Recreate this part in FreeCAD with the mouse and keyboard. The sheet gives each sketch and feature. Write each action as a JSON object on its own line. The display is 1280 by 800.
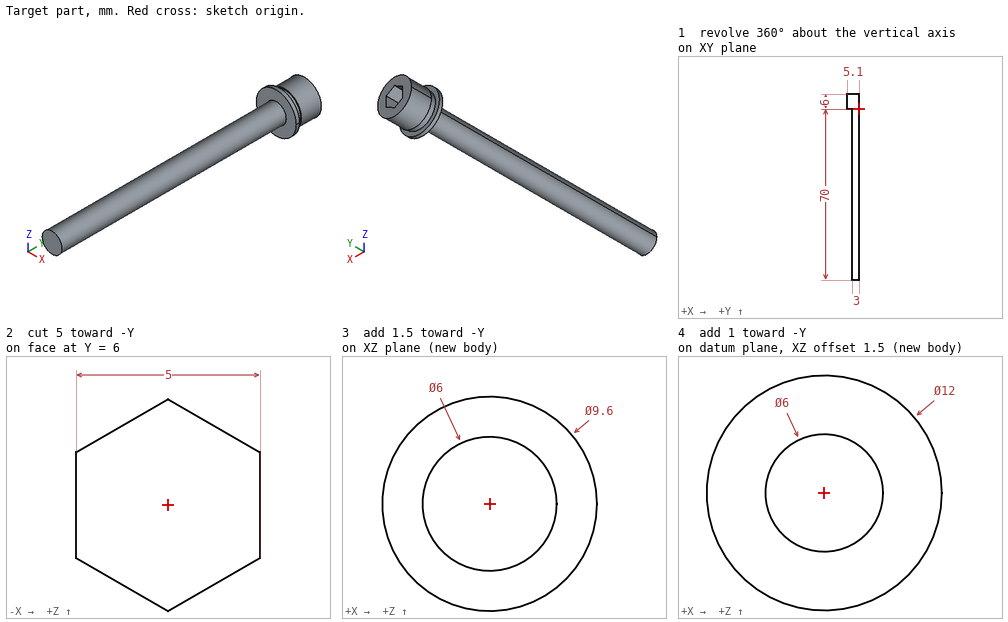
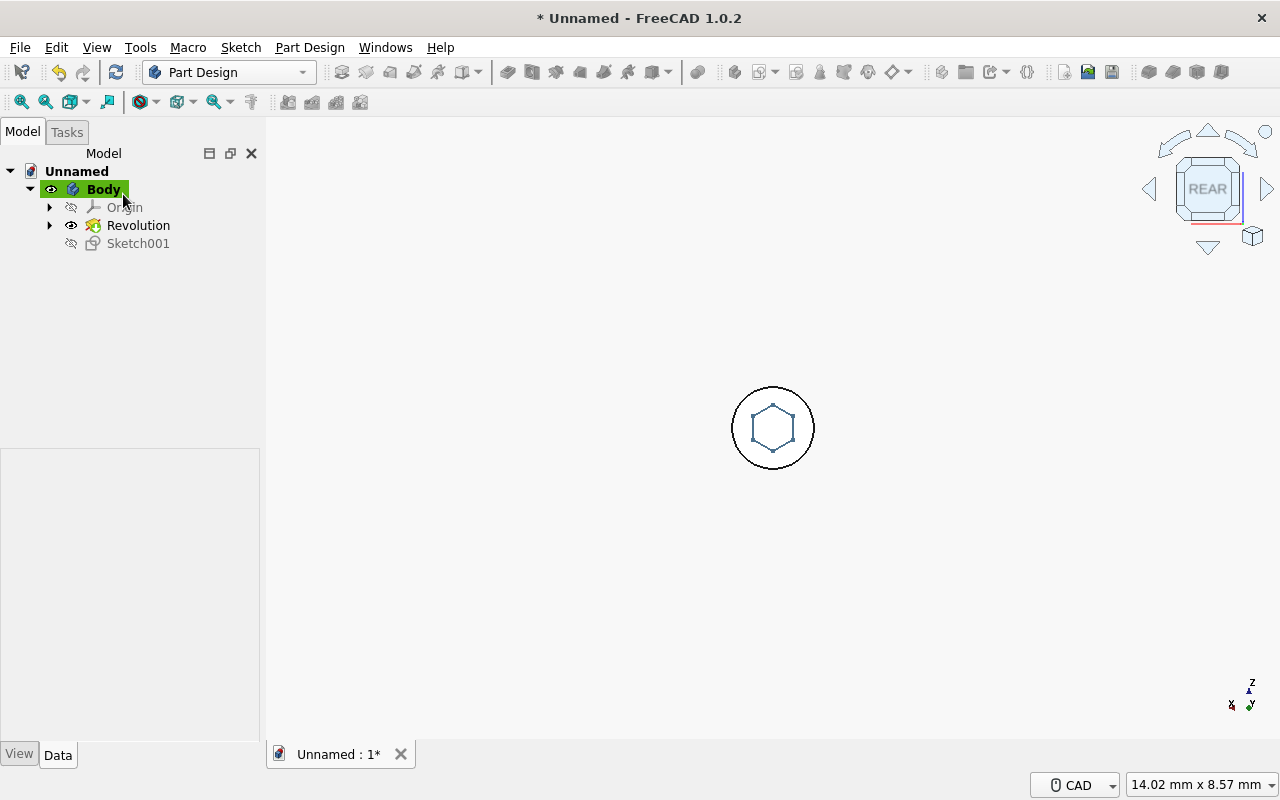
{"action": "left_click", "coordinate": [508, 72]}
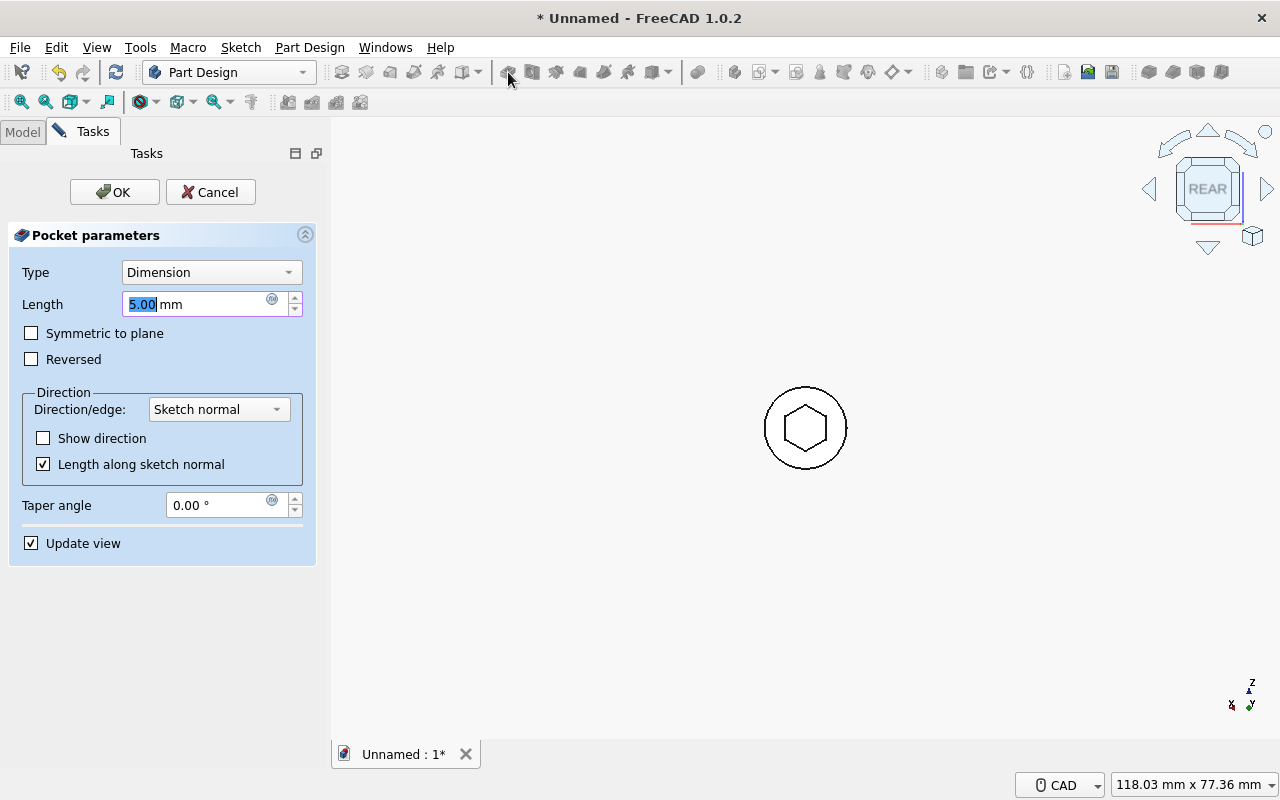
{"action": "type", "text": "5"}
{"action": "key", "text": "Tab"}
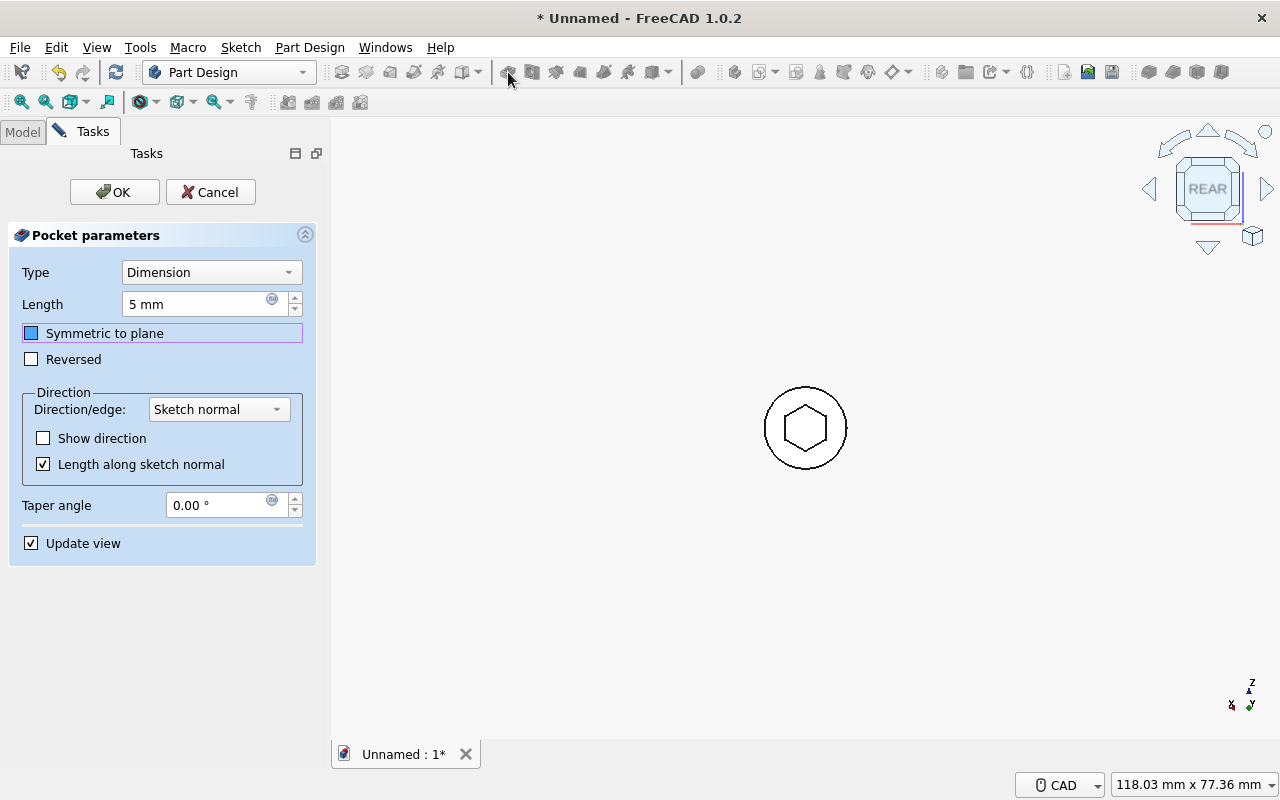
{"action": "left_click", "coordinate": [115, 192]}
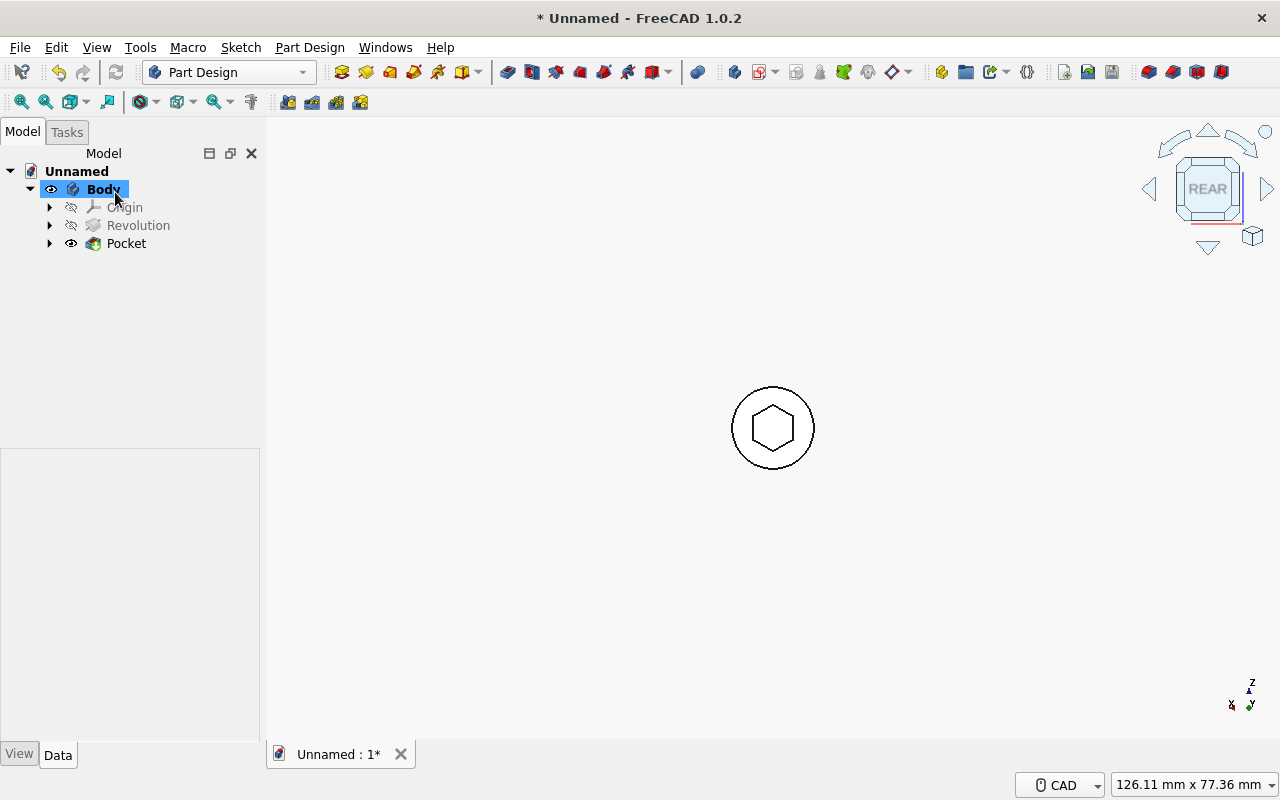
{"action": "key", "text": "v f"}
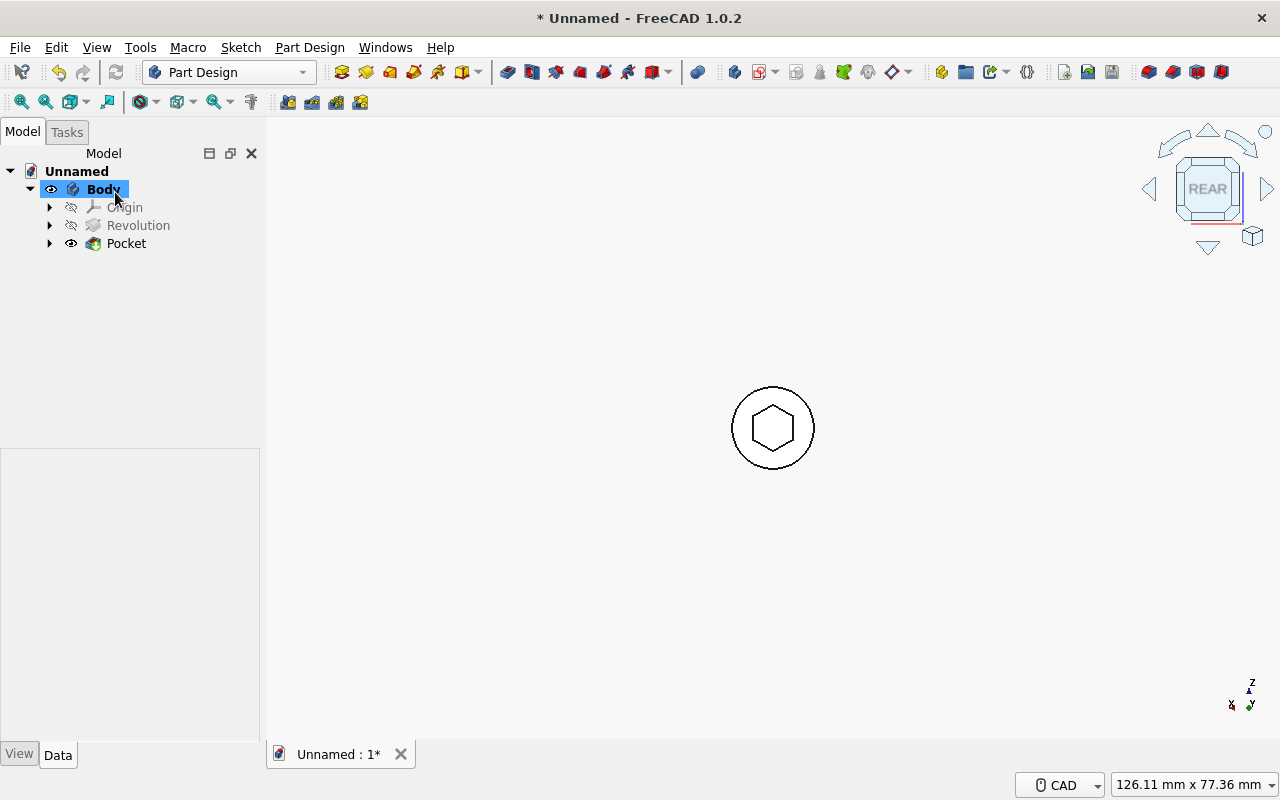
{"action": "left_click", "coordinate": [736, 72]}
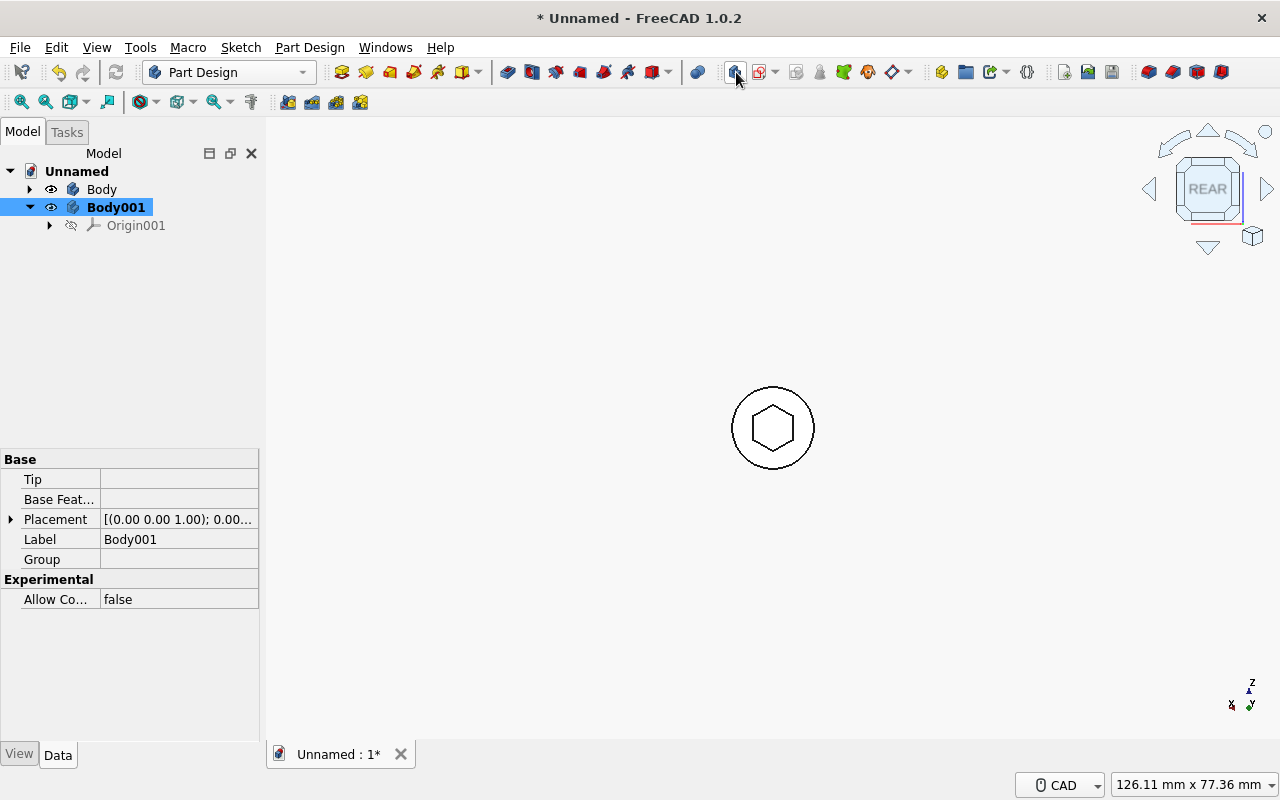
{"action": "left_click", "coordinate": [306, 699]}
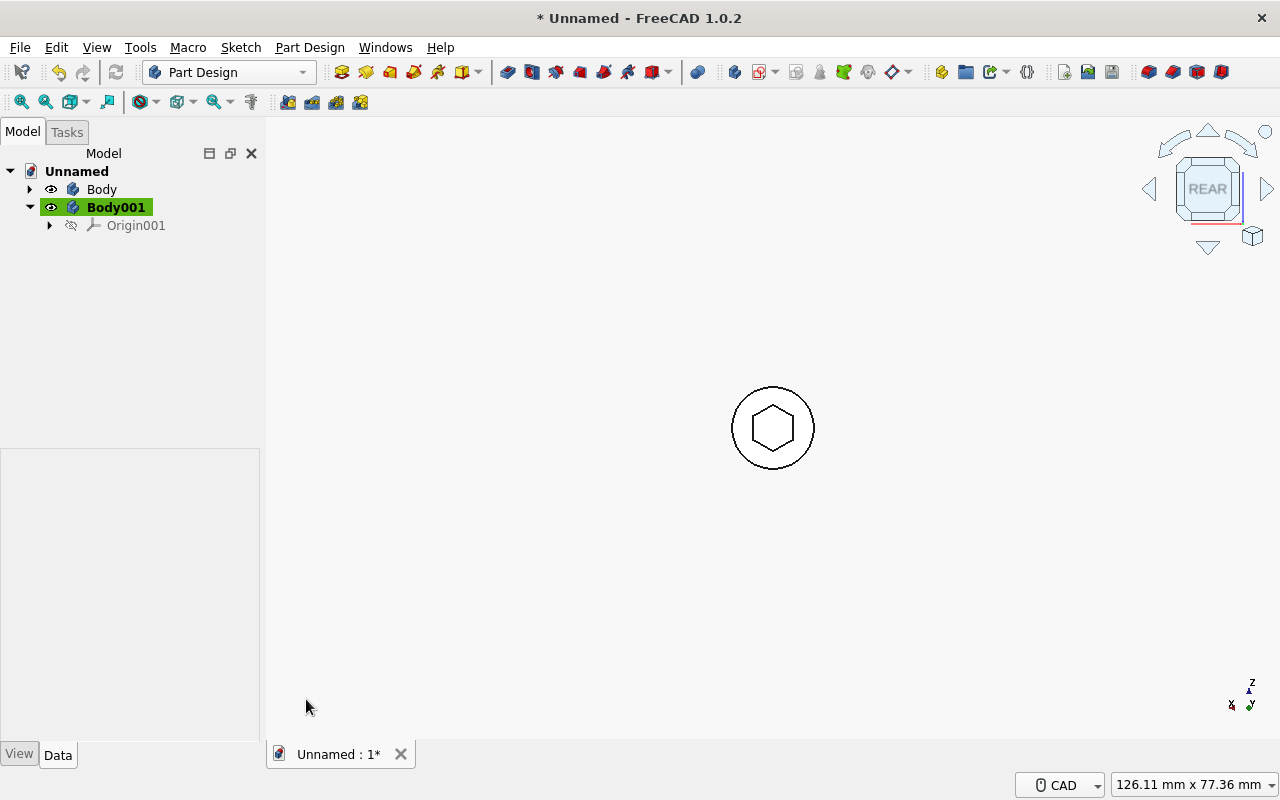
{"action": "left_click", "coordinate": [760, 72]}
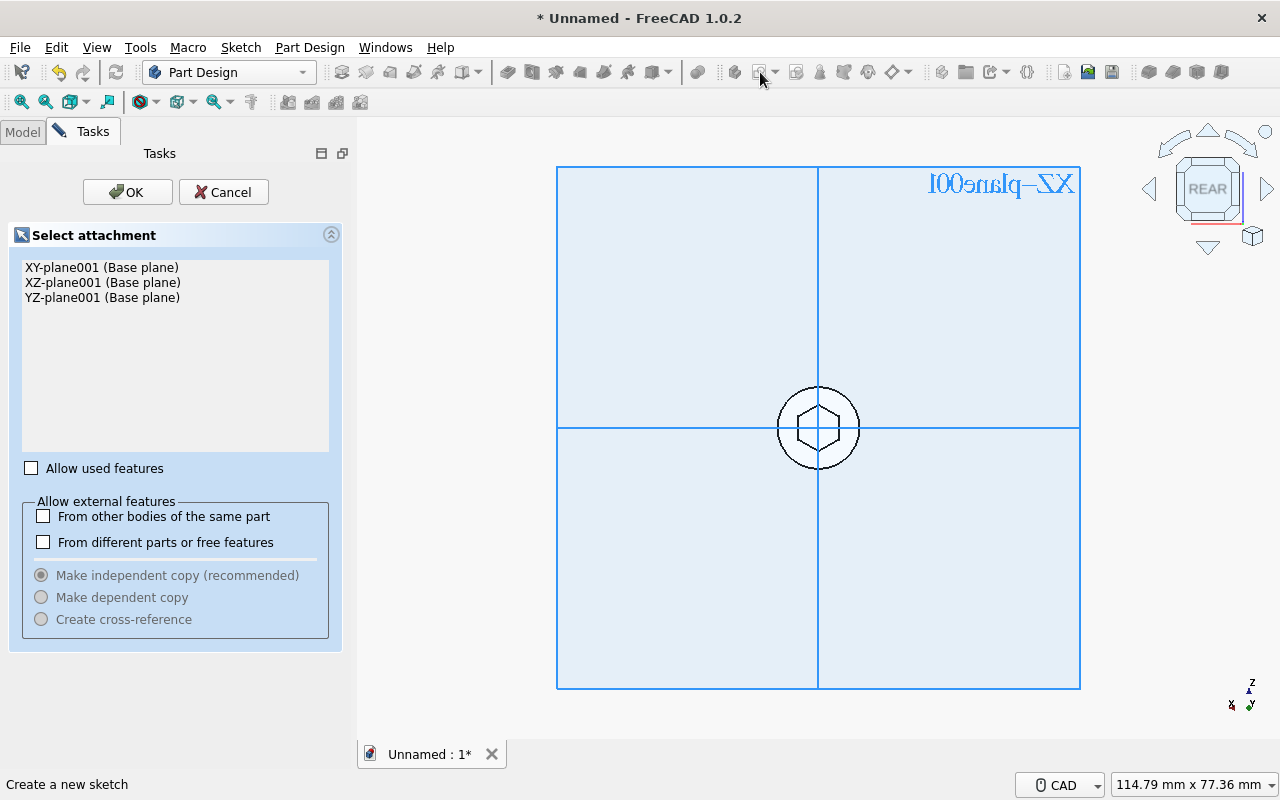
{"action": "left_click", "coordinate": [82, 282]}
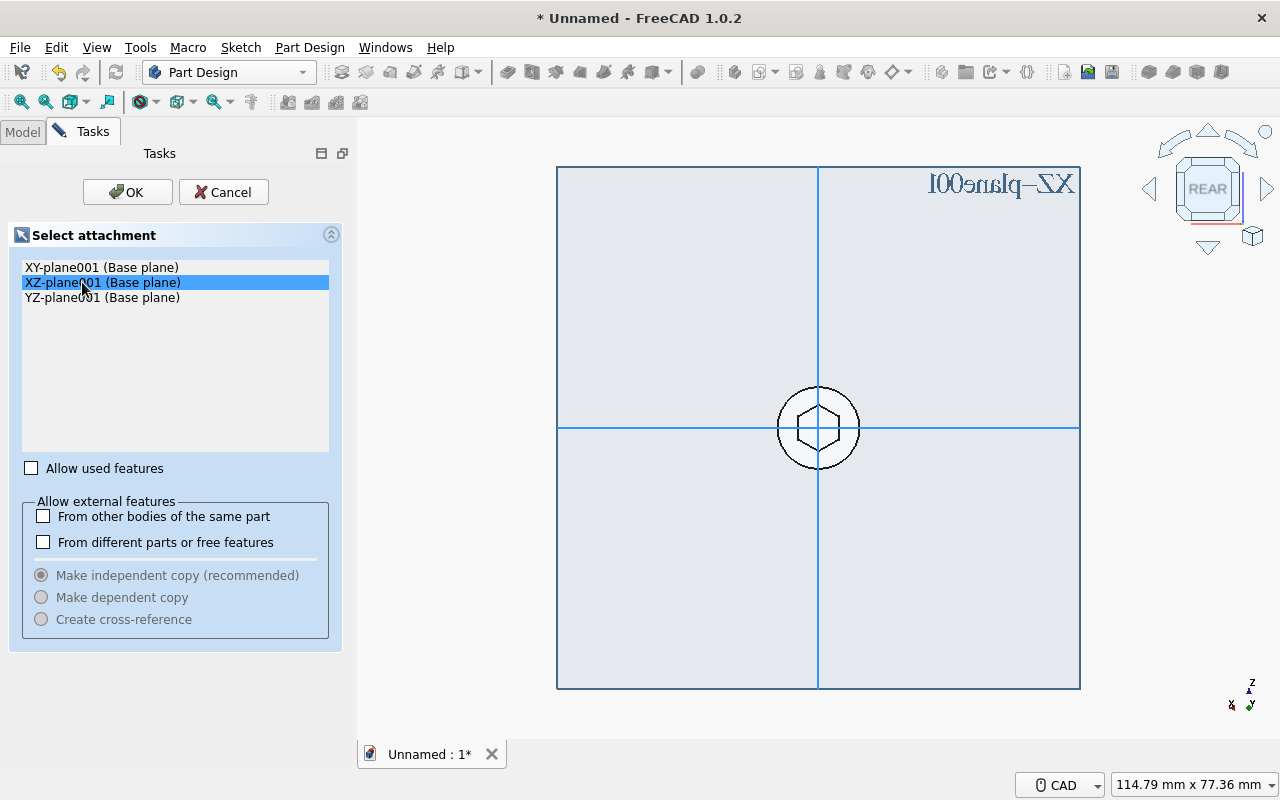
{"action": "left_click", "coordinate": [128, 192]}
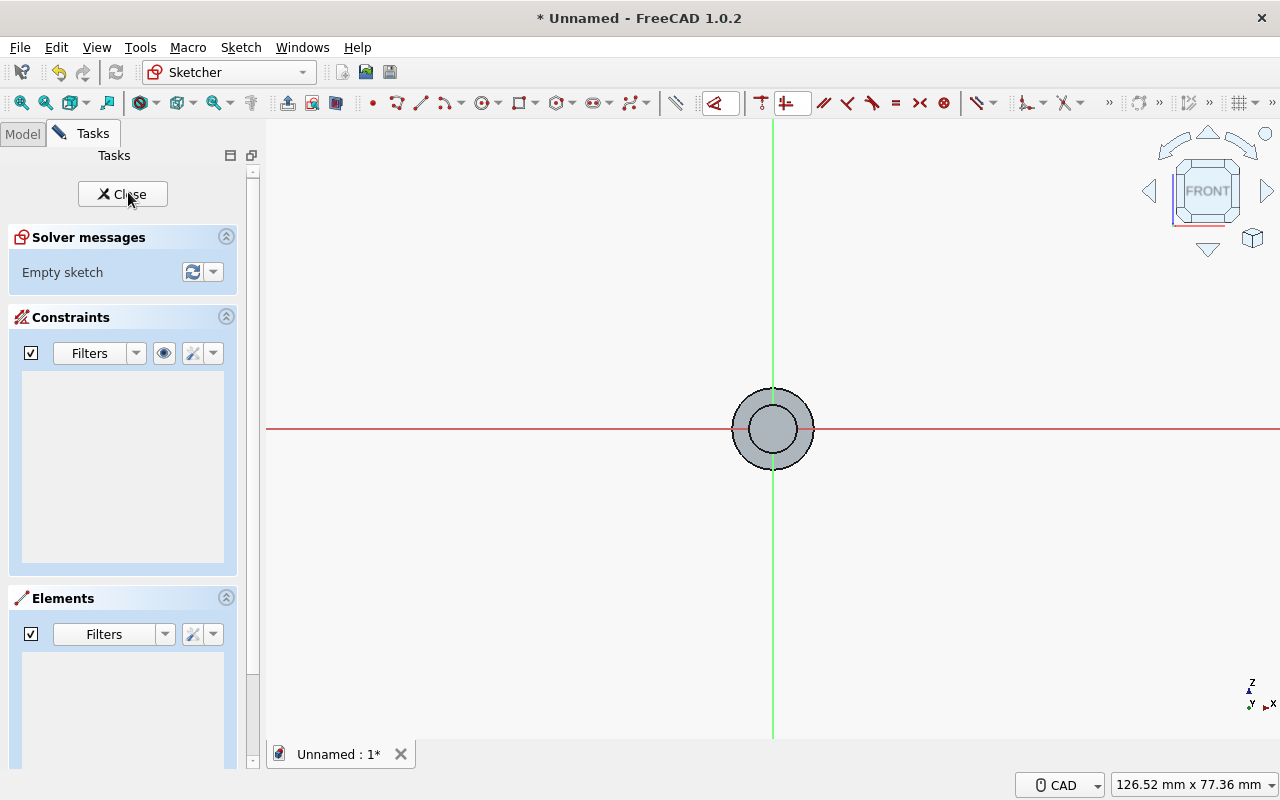
{"action": "scroll", "coordinate": [790, 429], "scroll_direction": "up", "scroll_amount": 8}